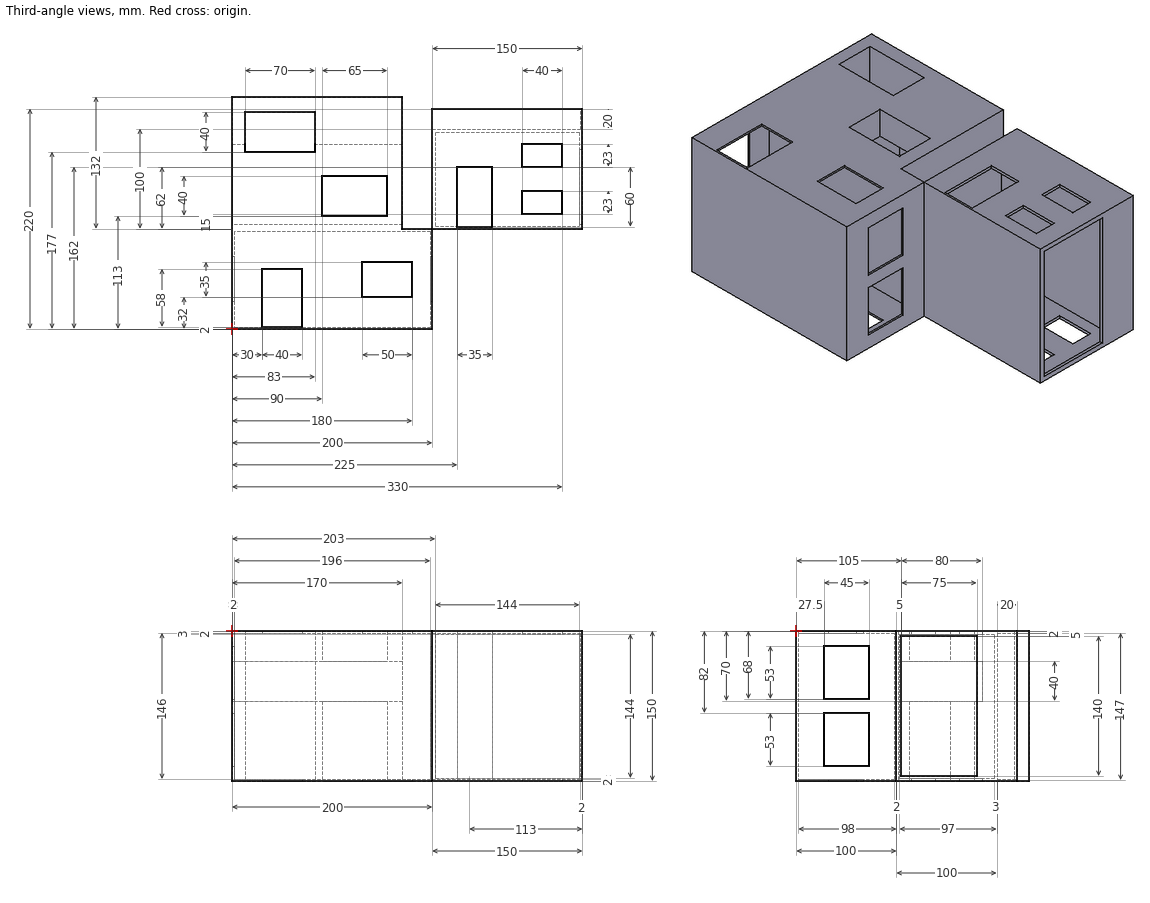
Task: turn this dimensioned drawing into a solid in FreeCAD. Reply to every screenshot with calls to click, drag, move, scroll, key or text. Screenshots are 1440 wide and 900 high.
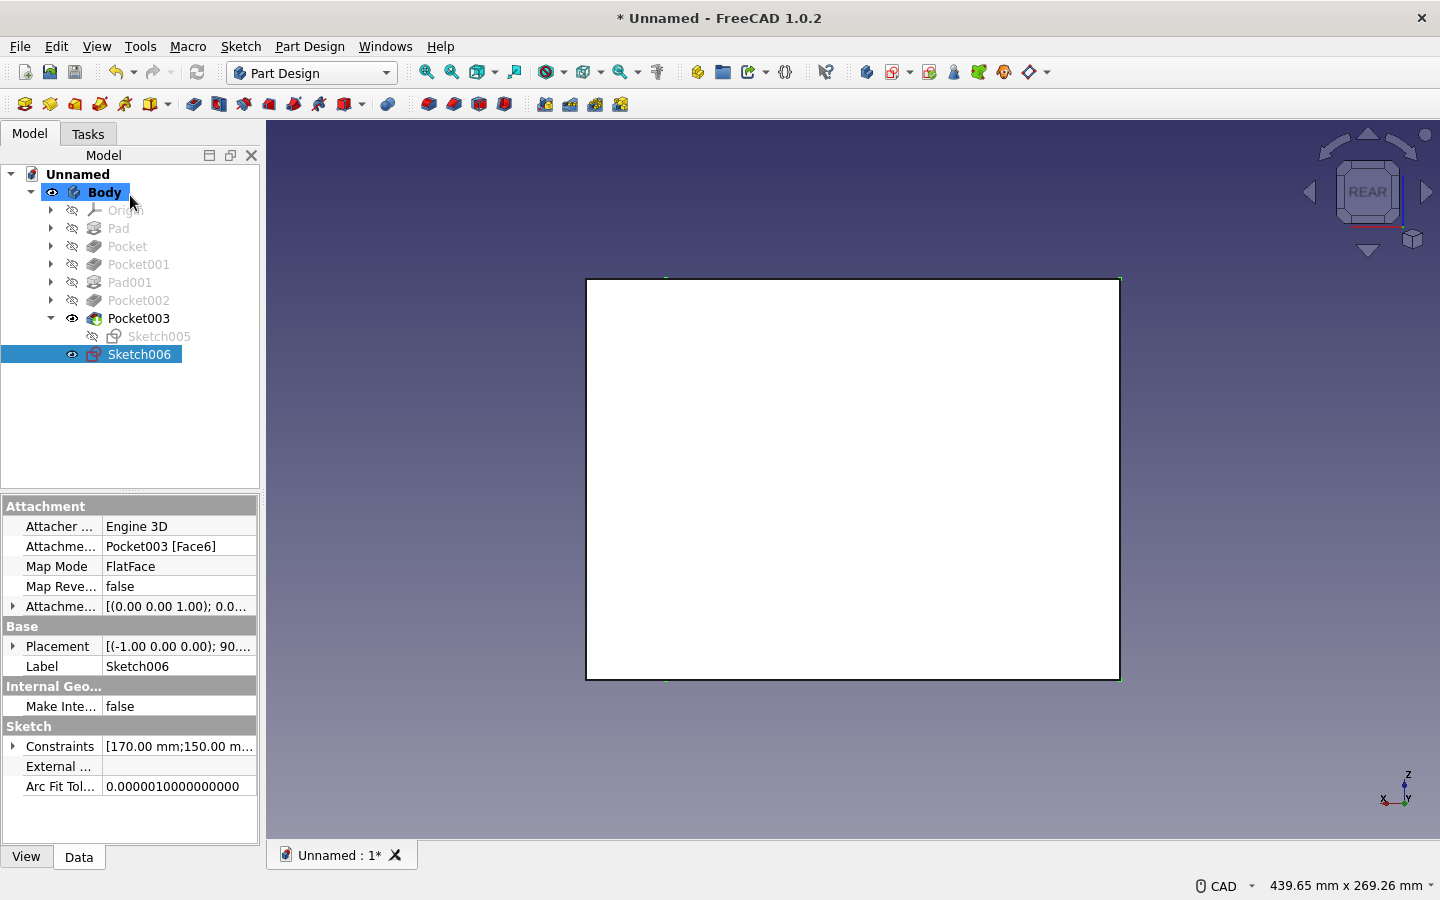
click(25, 104)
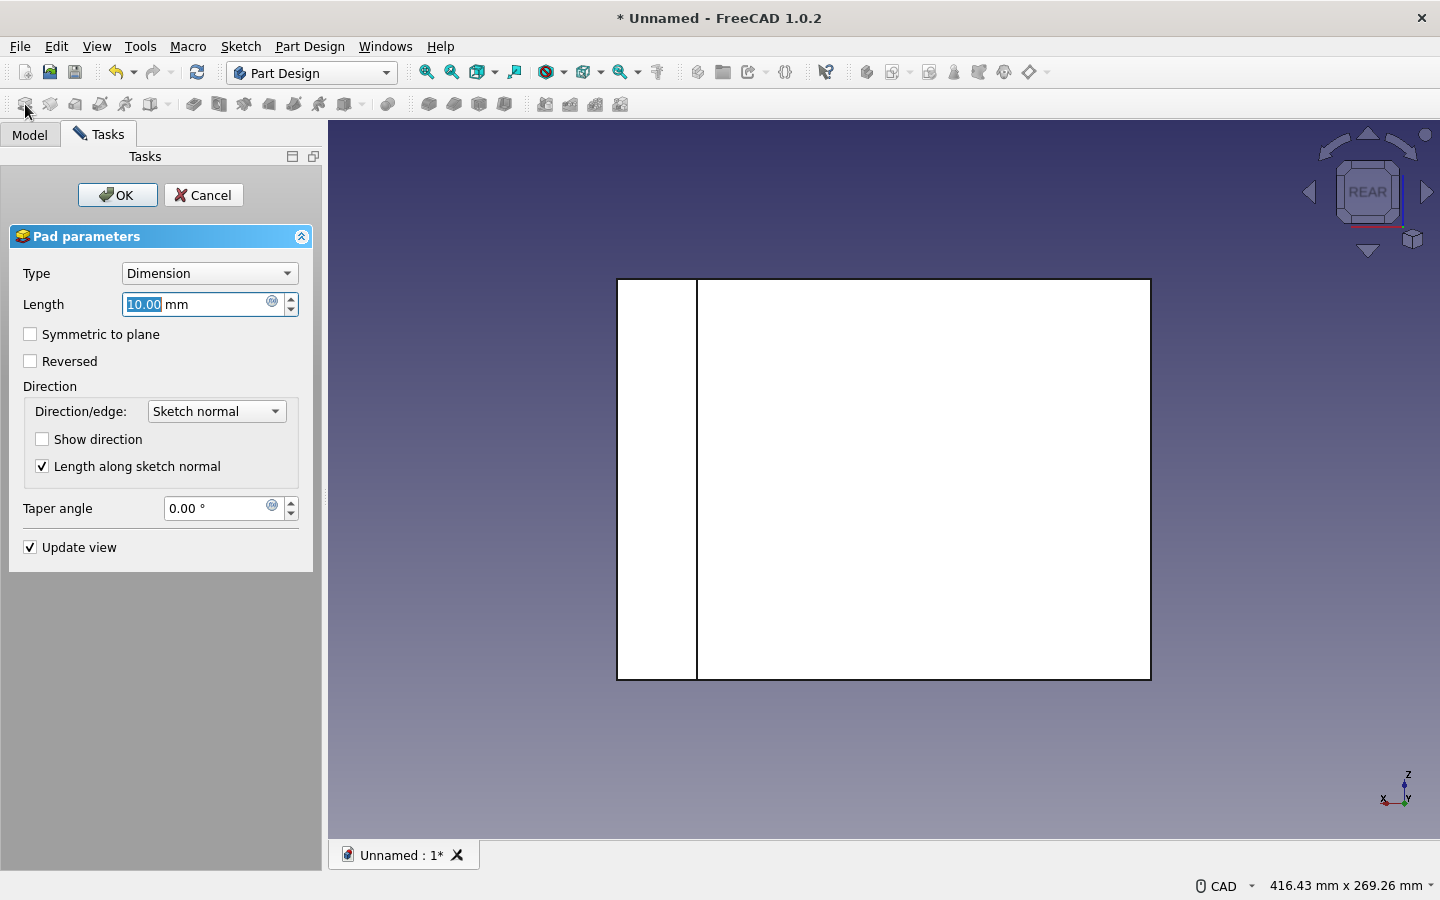
text(132)
key(Tab)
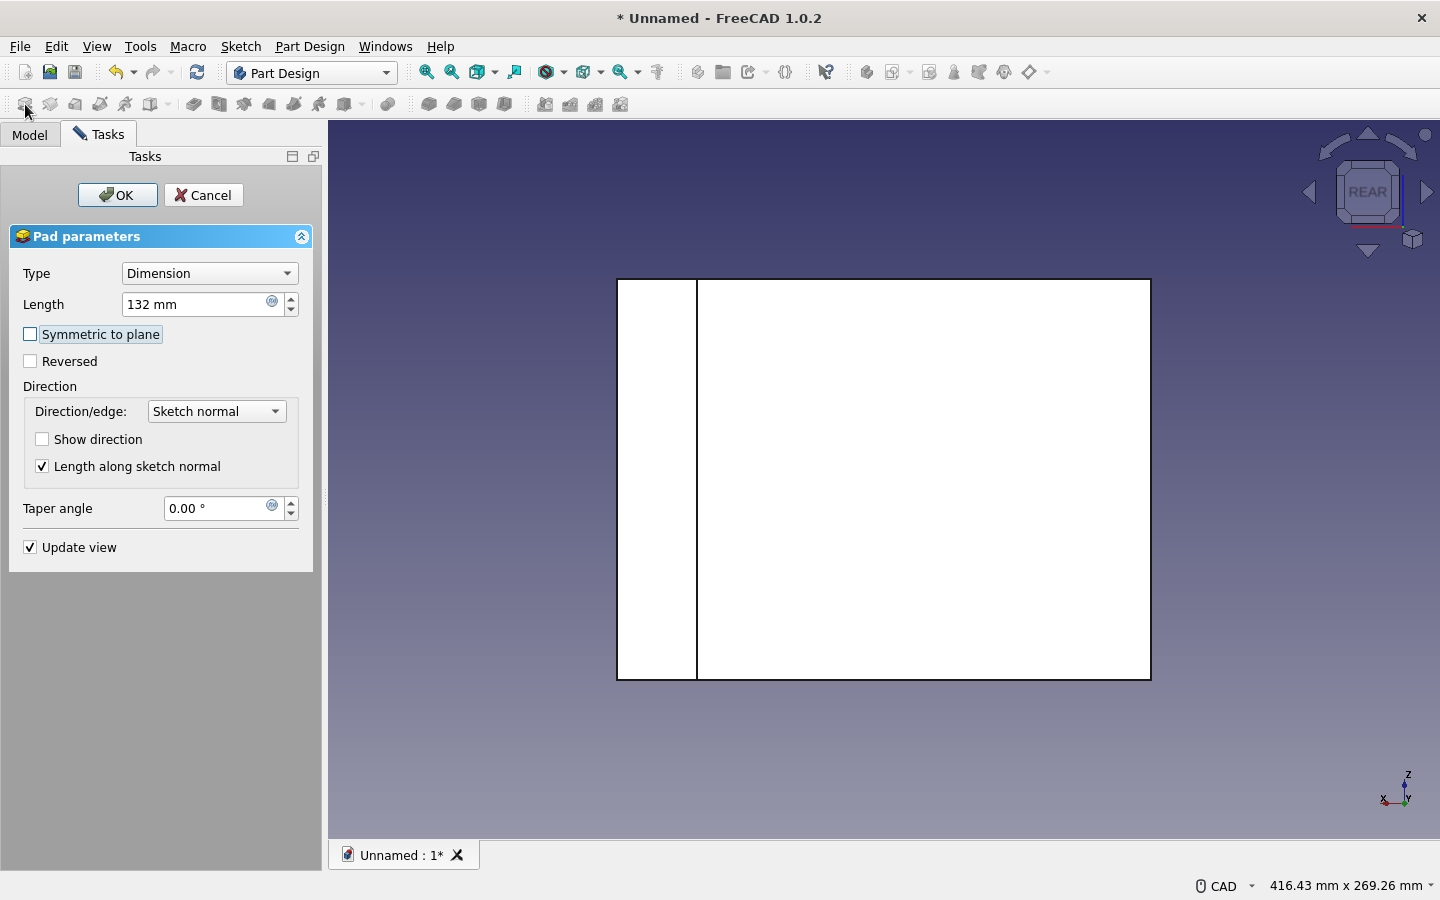
click(118, 195)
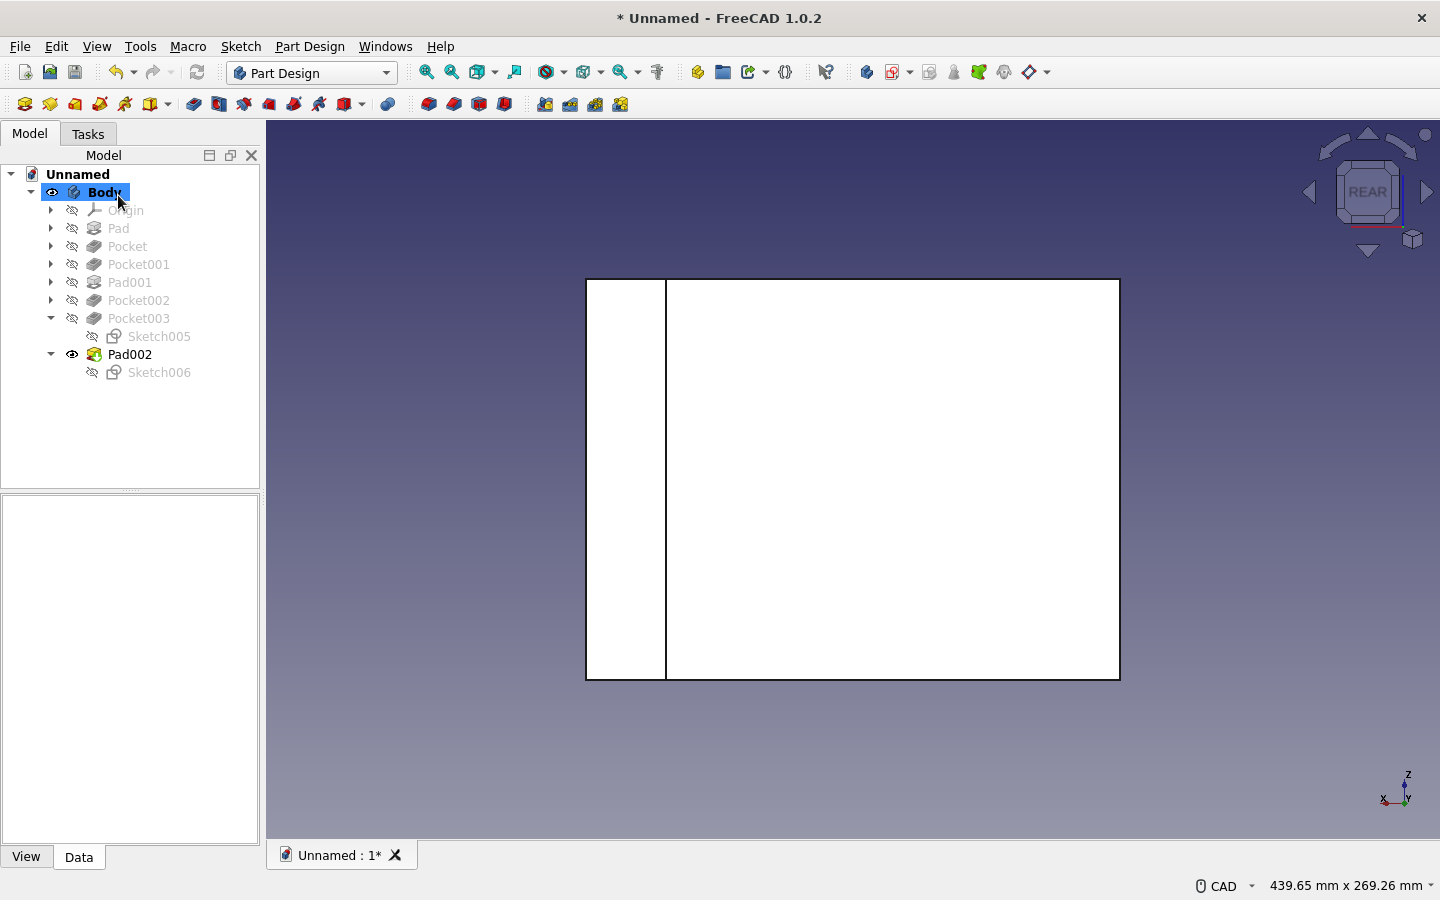
key(0)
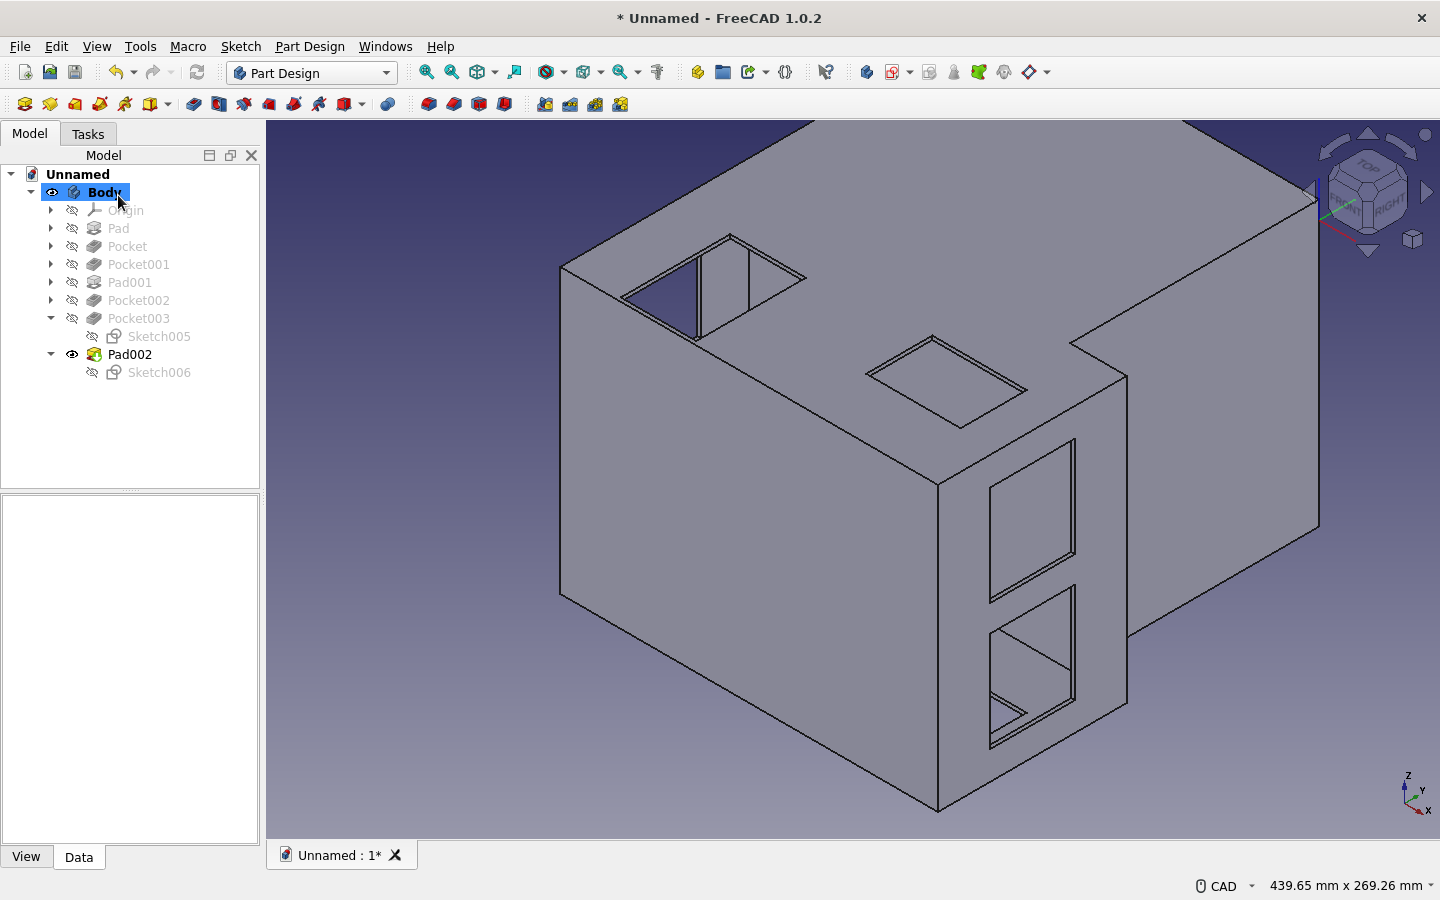
click(427, 72)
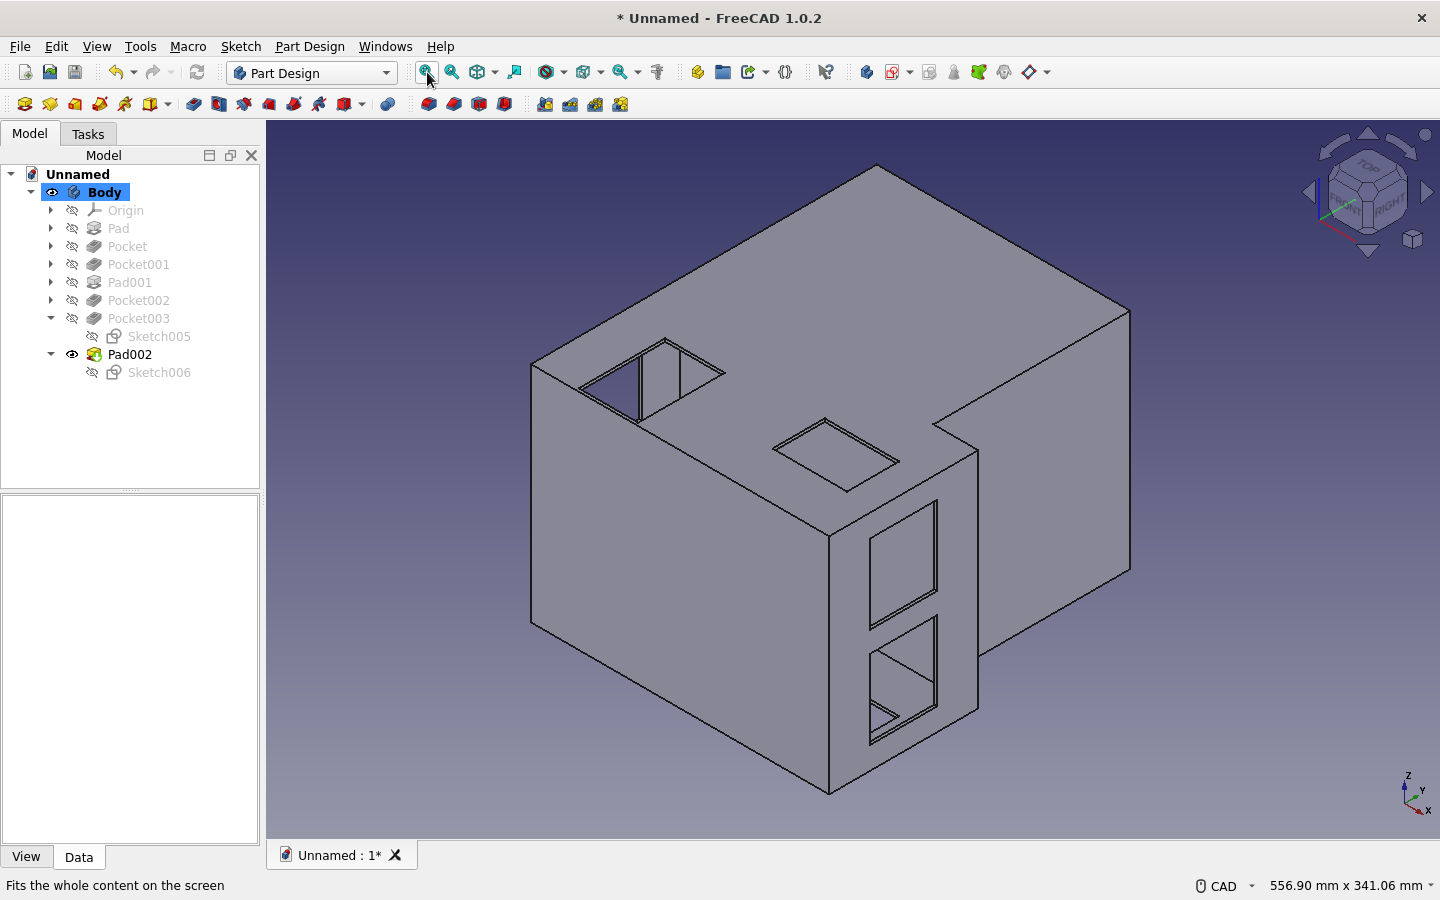
click(860, 296)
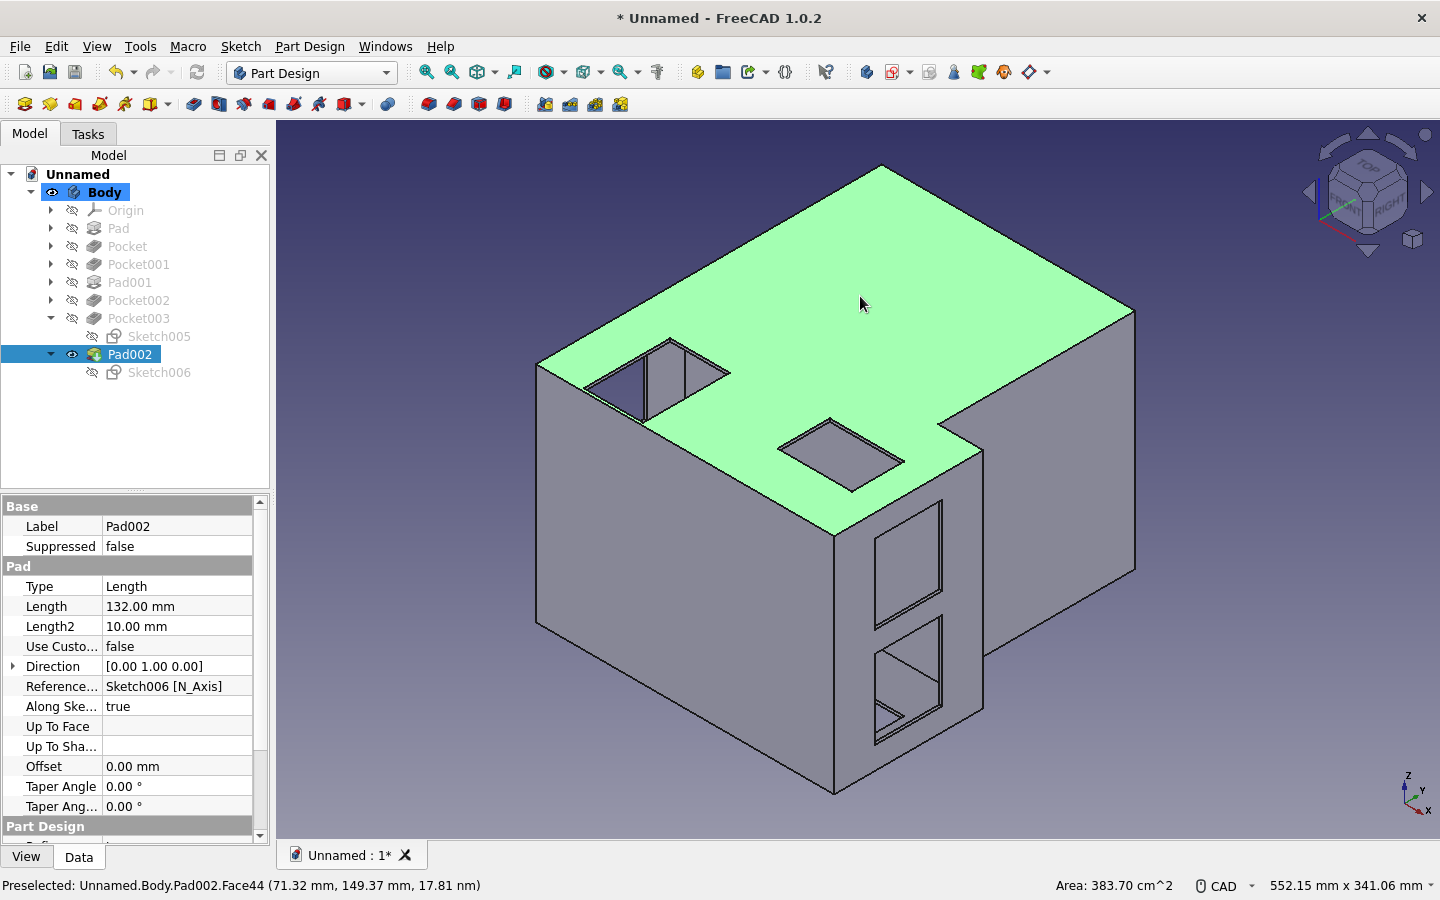
click(892, 72)